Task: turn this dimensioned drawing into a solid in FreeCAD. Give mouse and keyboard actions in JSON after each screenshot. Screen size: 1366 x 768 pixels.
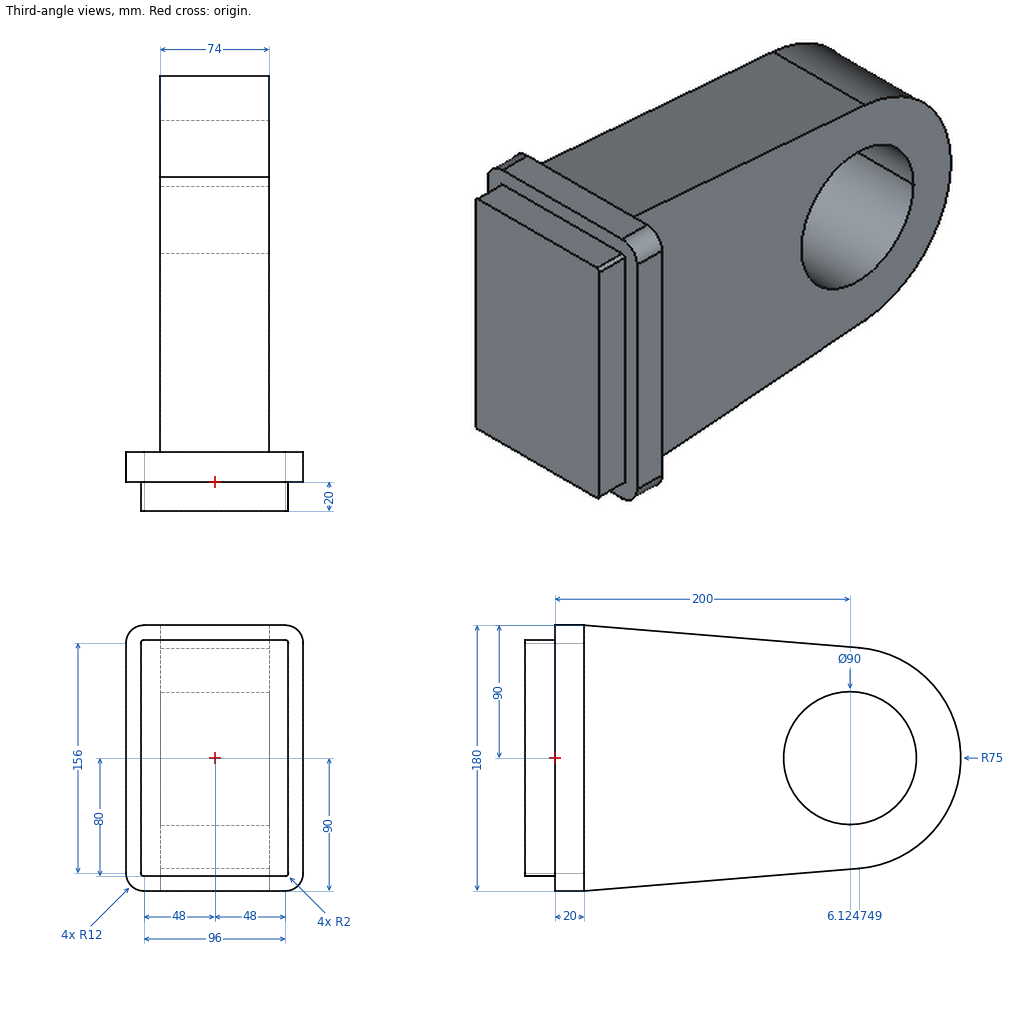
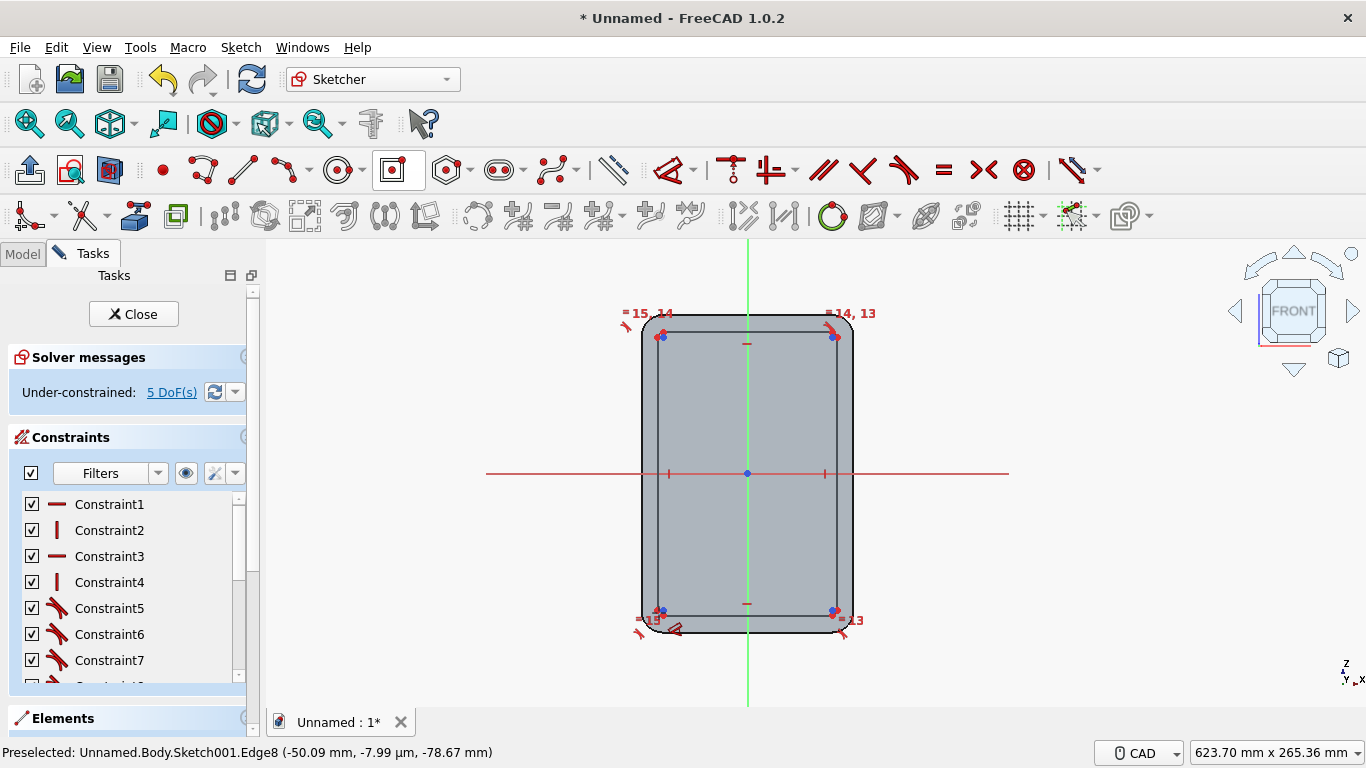
{"action": "scroll", "coordinate": [834, 615], "scroll_direction": "up", "scroll_amount": 13}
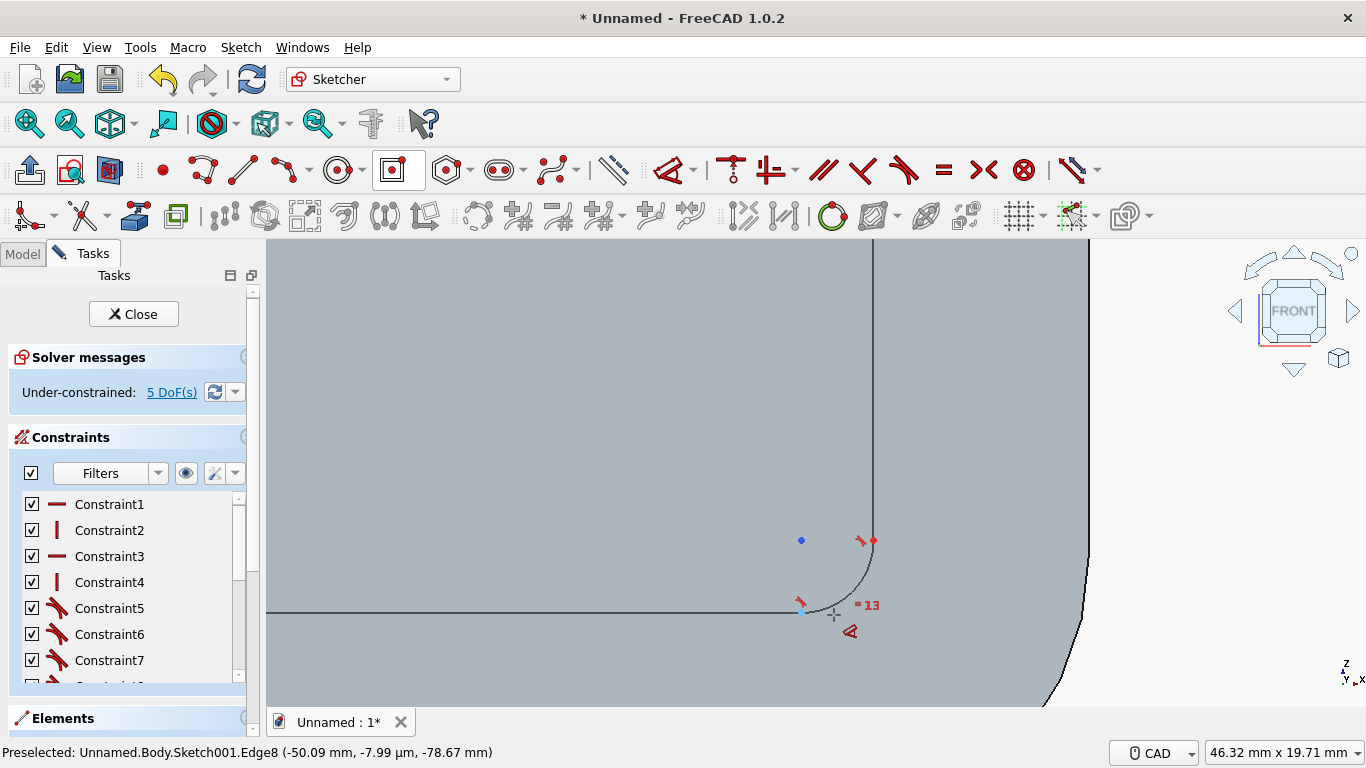
{"action": "left_click", "coordinate": [834, 605]}
{"action": "left_click", "coordinate": [848, 634]}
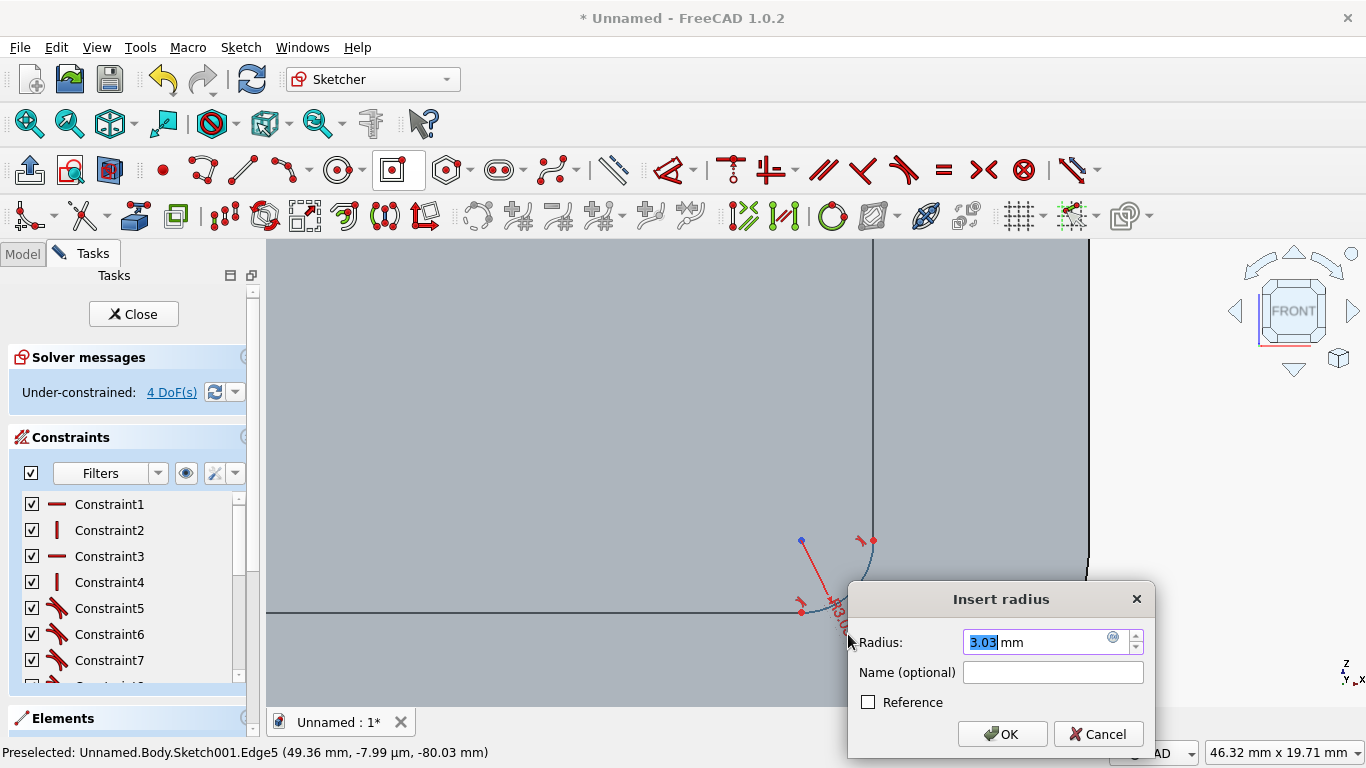
{"action": "type", "text": "2"}
{"action": "key", "text": "Return"}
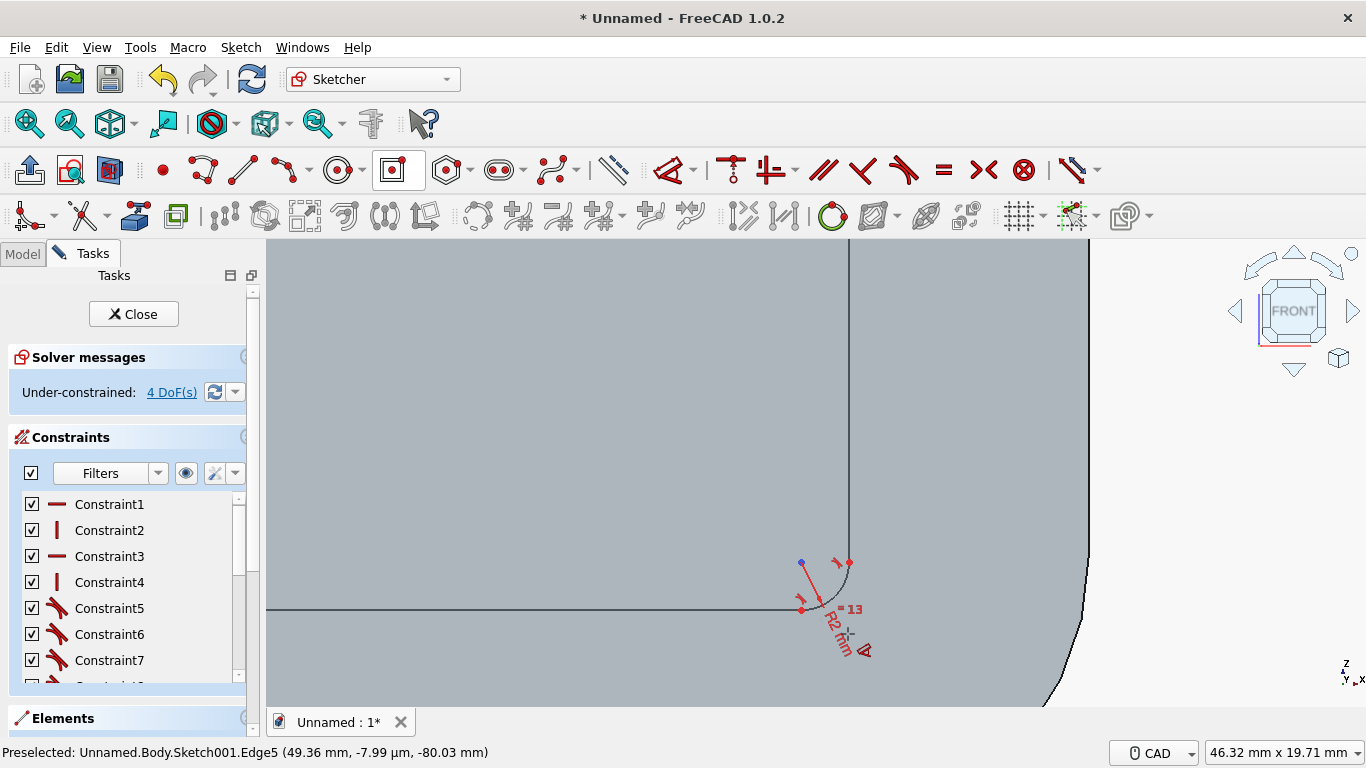
{"action": "scroll", "coordinate": [834, 615], "scroll_direction": "down", "scroll_amount": 13}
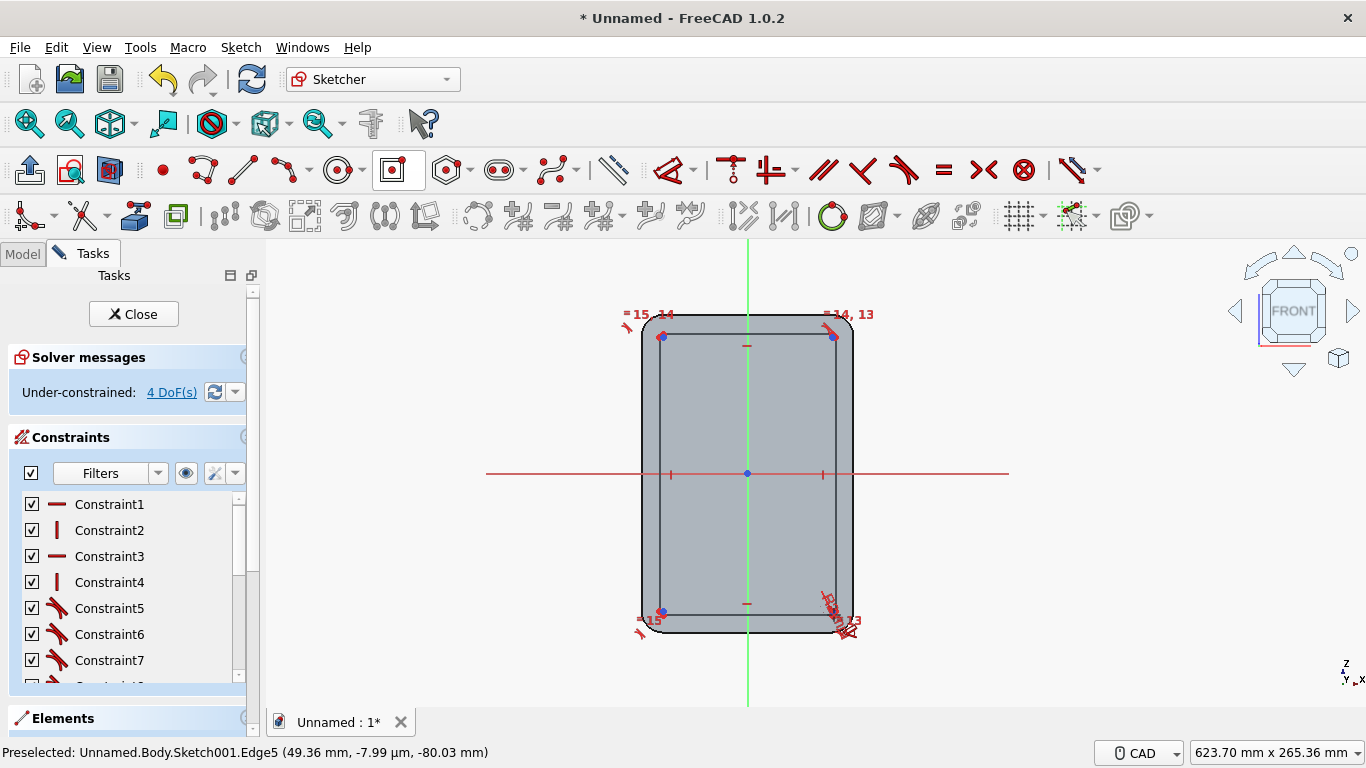
{"action": "left_click", "coordinate": [798, 615]}
{"action": "left_click", "coordinate": [709, 649]}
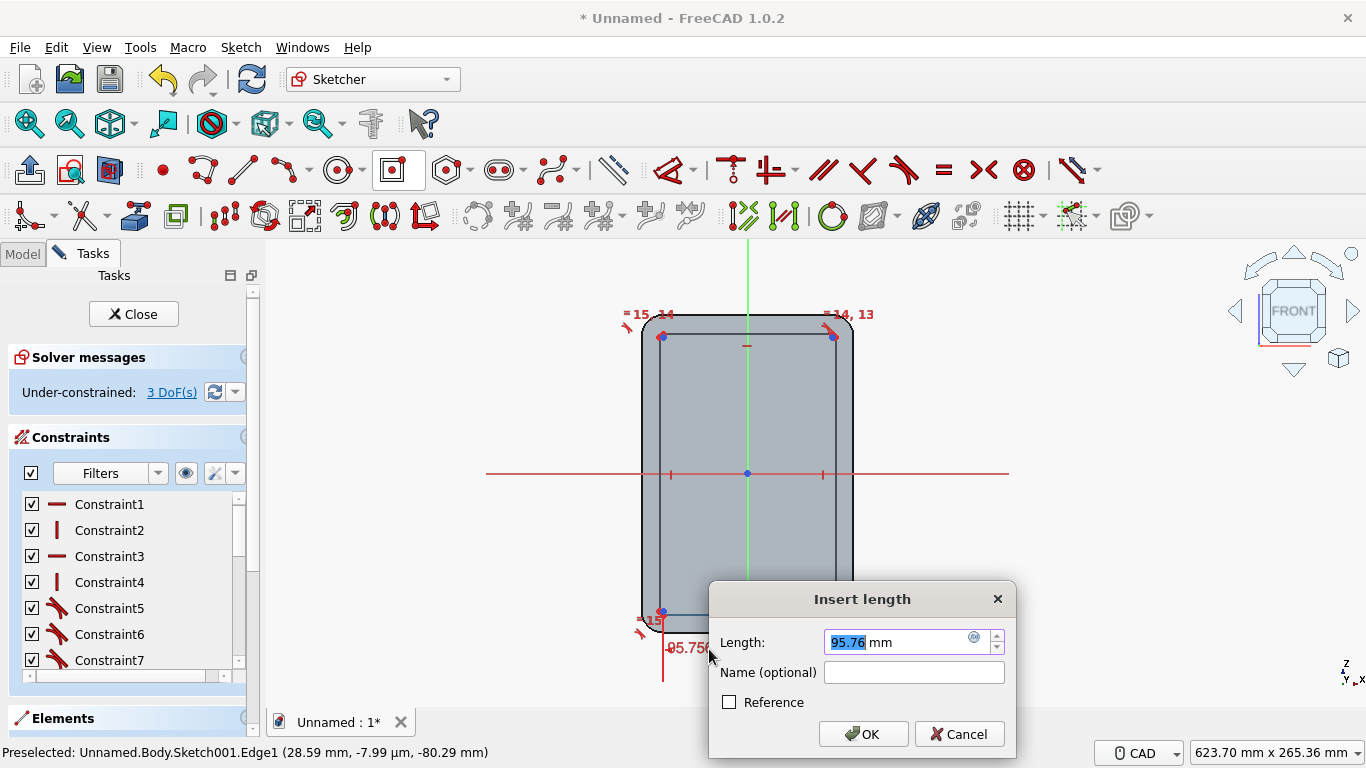
{"action": "type", "text": "96"}
{"action": "key", "text": "Return"}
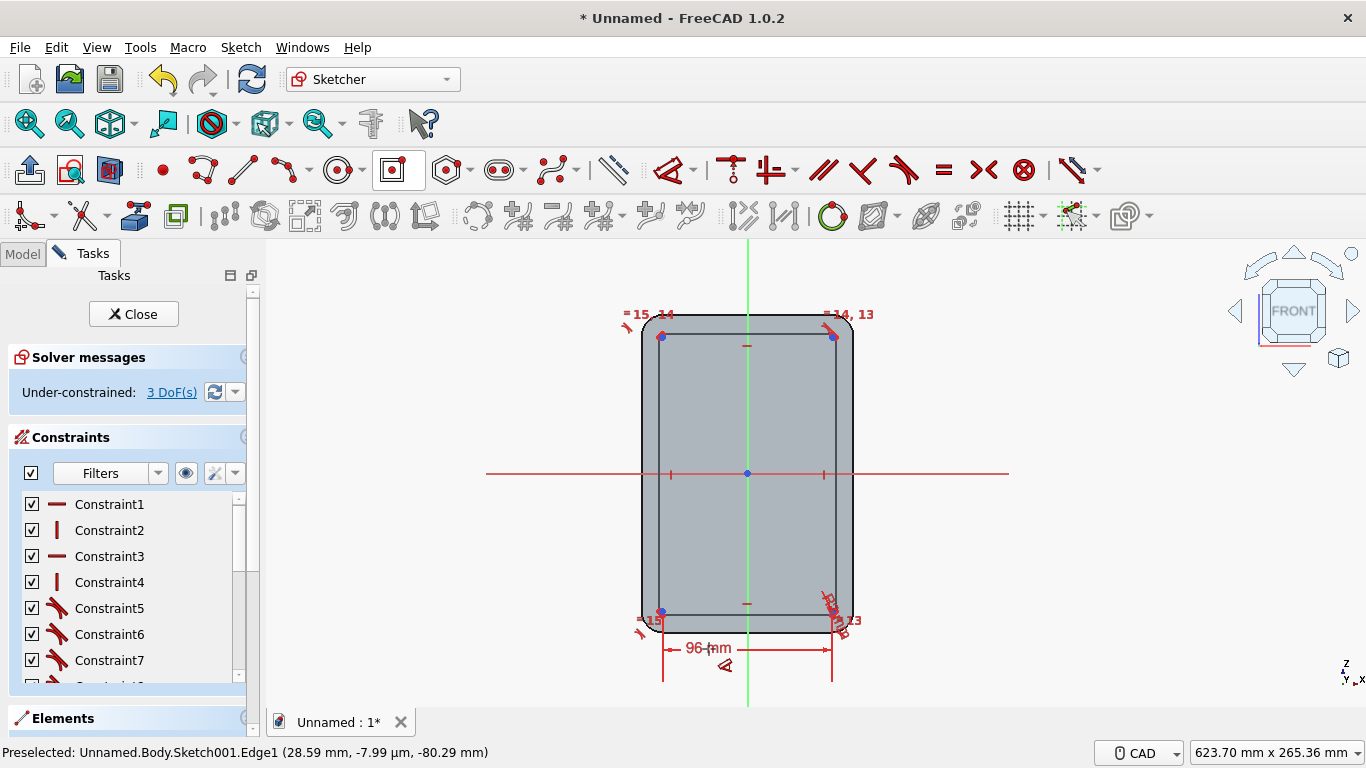
{"action": "left_click", "coordinate": [836, 530]}
{"action": "left_click", "coordinate": [870, 412]}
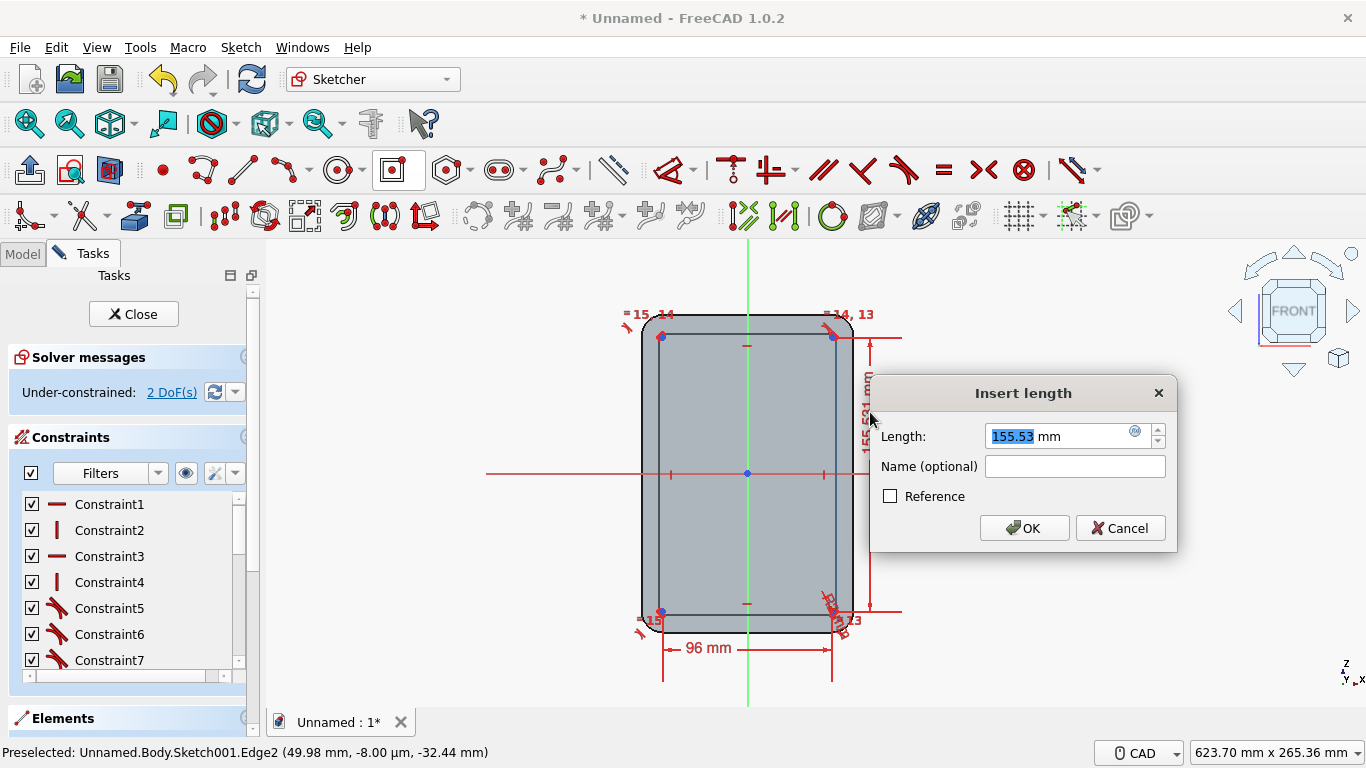
{"action": "type", "text": "156"}
{"action": "key", "text": "Return"}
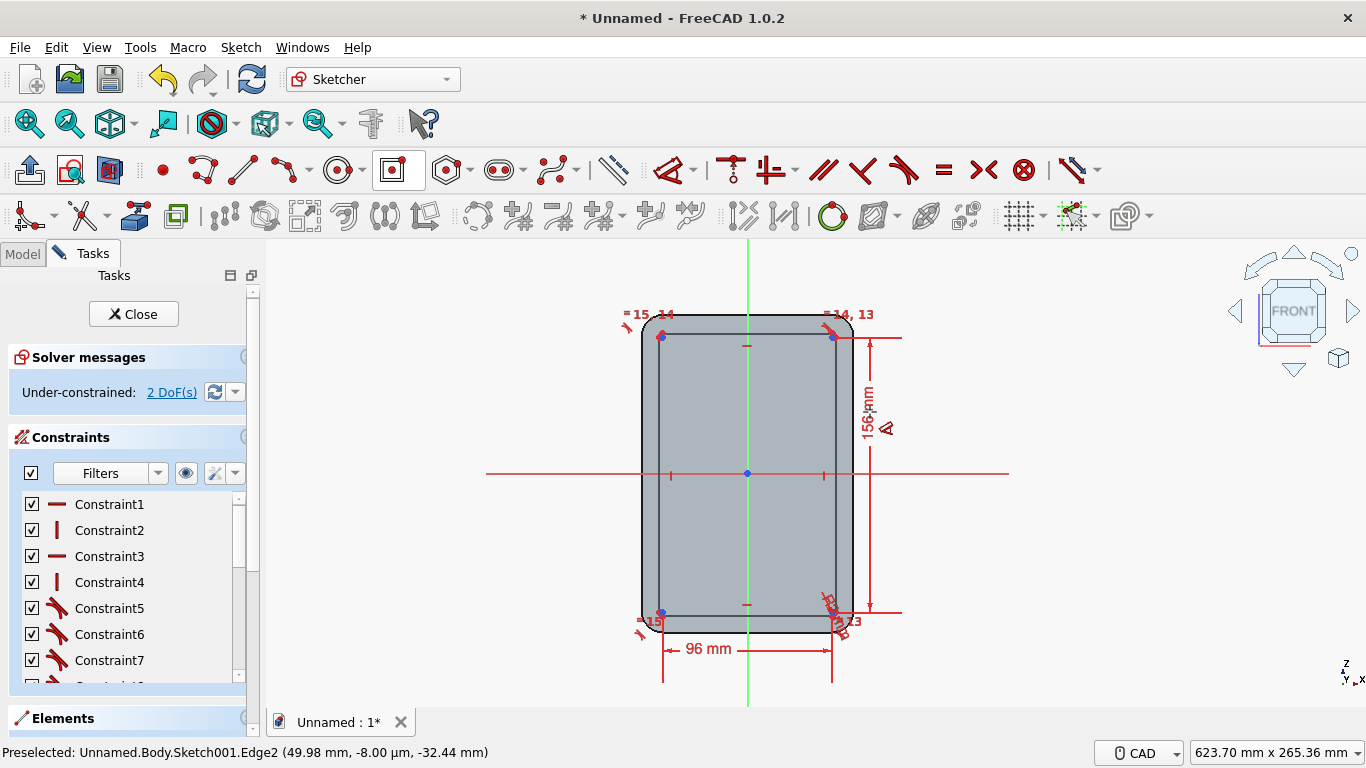
{"action": "scroll", "coordinate": [663, 616], "scroll_direction": "up", "scroll_amount": 7}